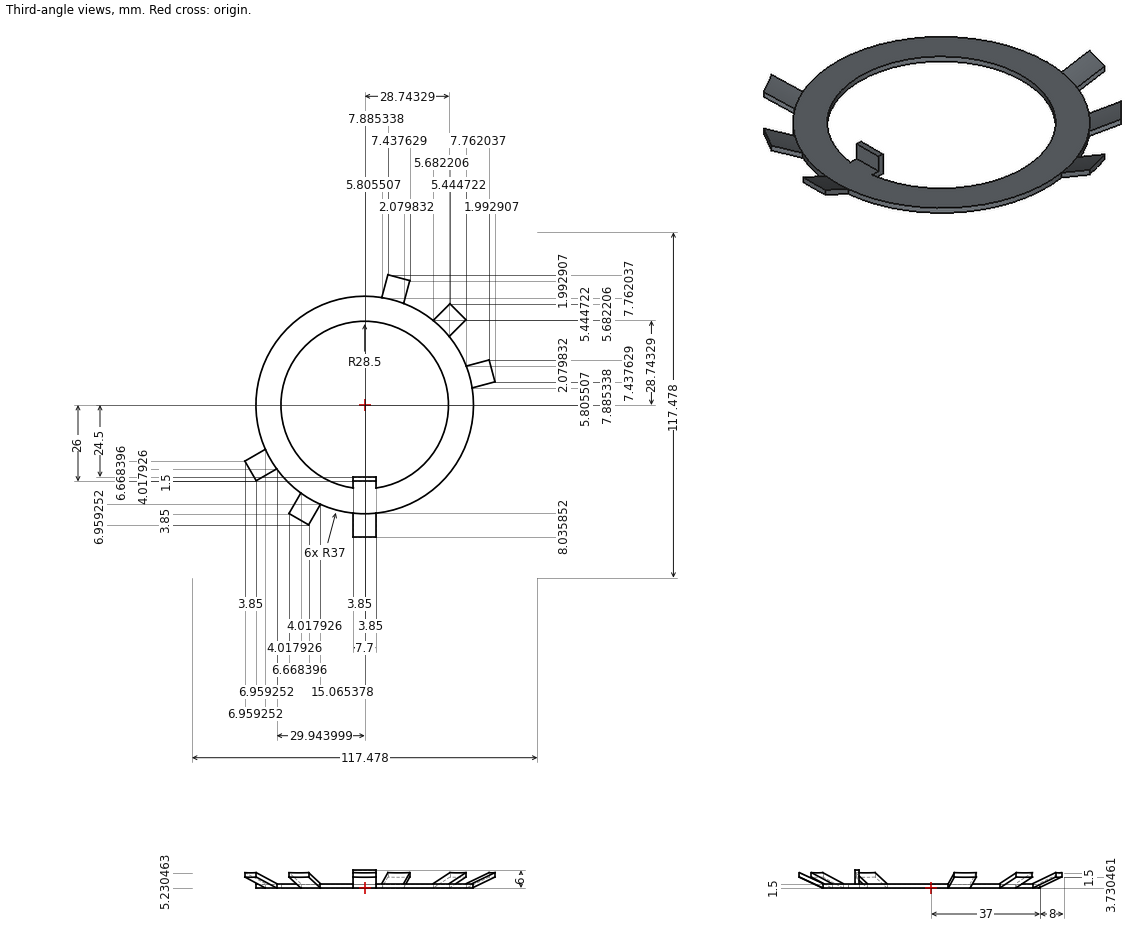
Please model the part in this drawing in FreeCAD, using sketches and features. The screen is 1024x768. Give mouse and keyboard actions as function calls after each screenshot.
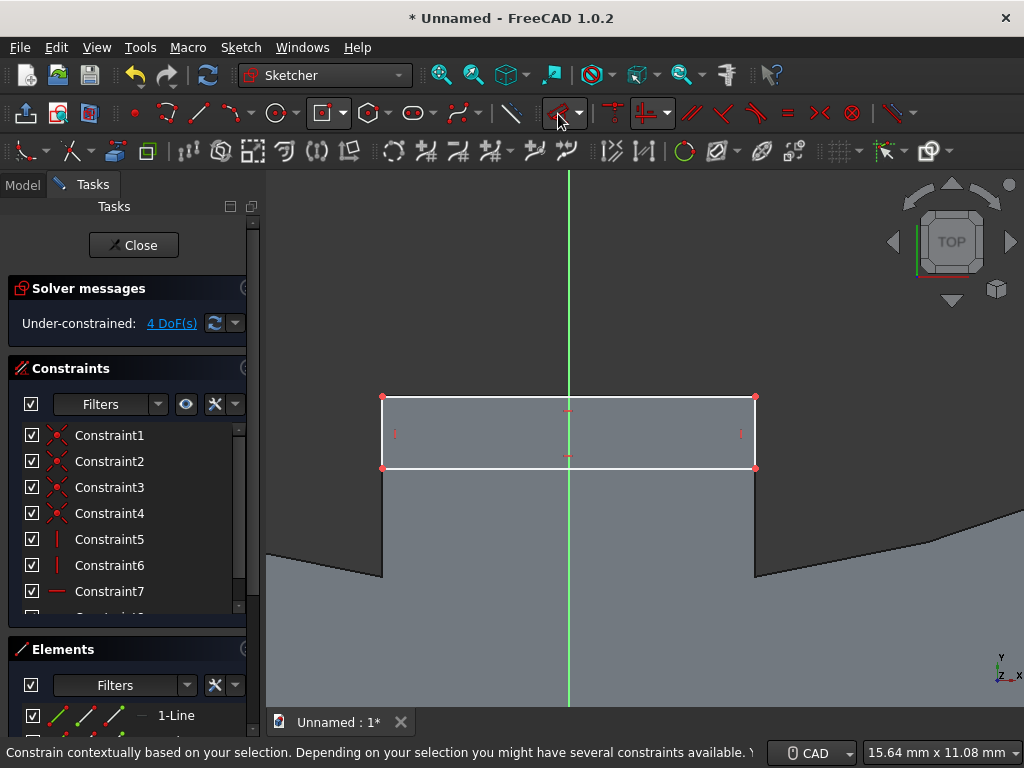
click(382, 419)
click(348, 433)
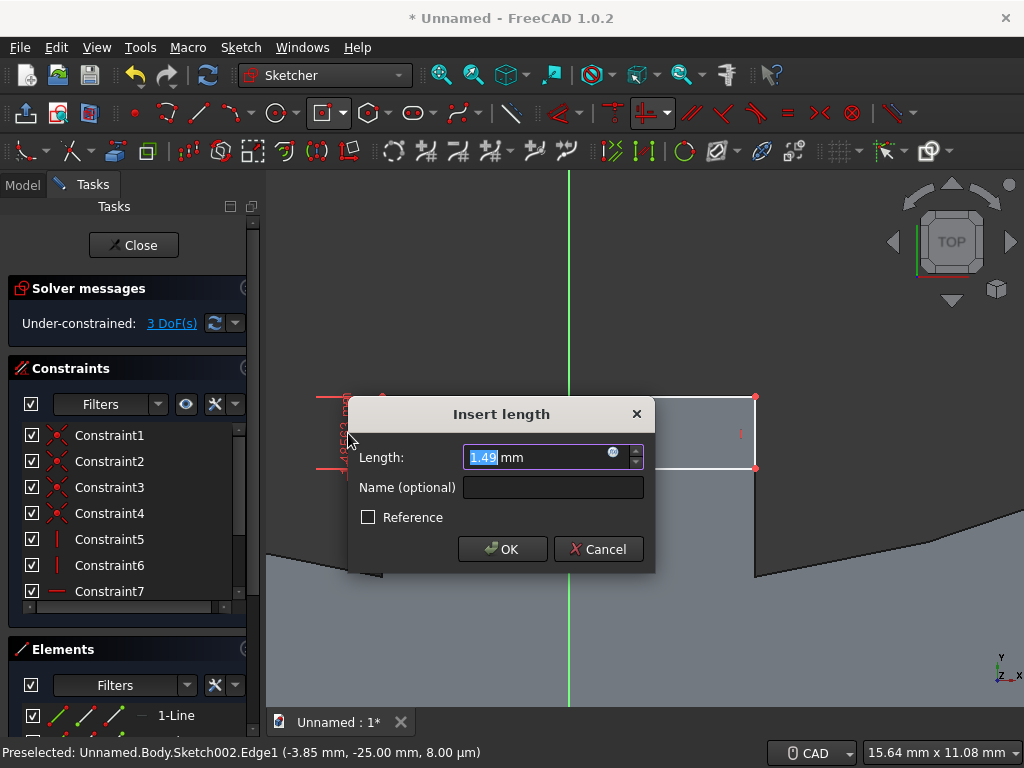
text(1.5)
key(Return)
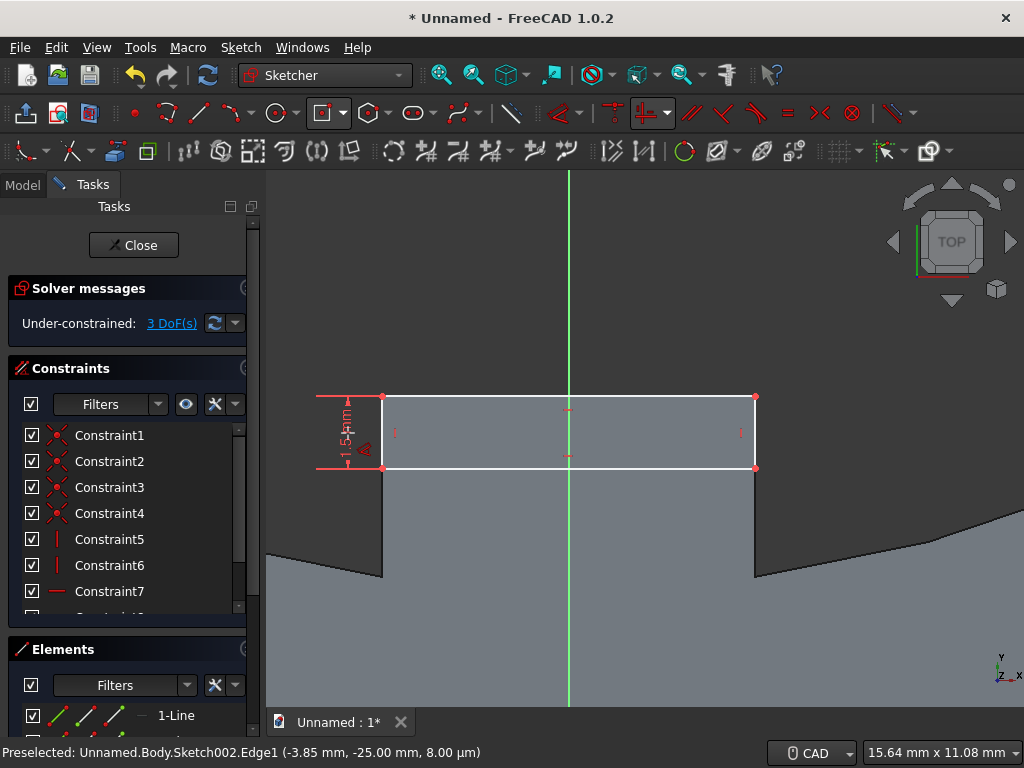
click(494, 469)
click(483, 503)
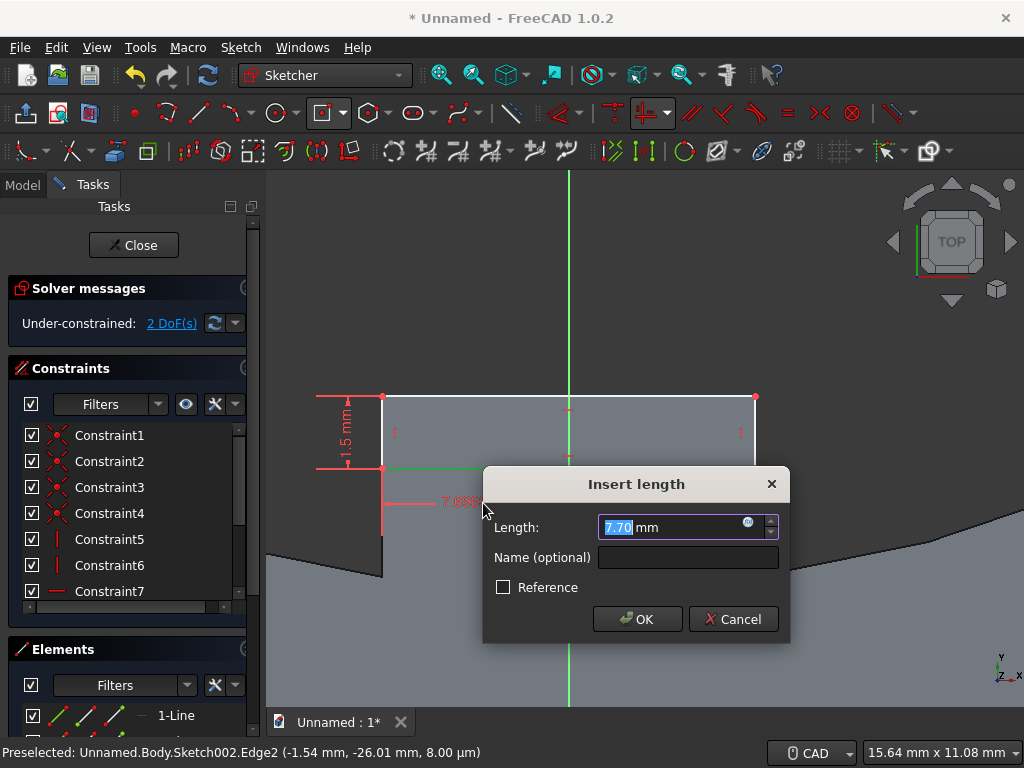
text(7.7)
key(Return)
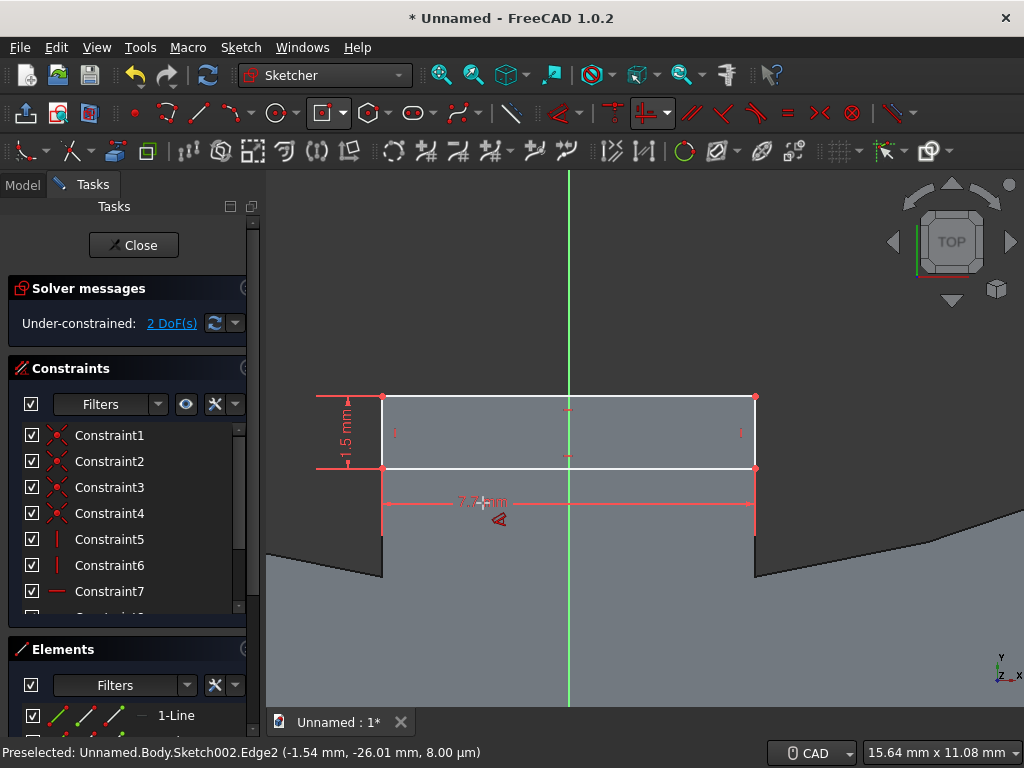
click(382, 469)
click(348, 334)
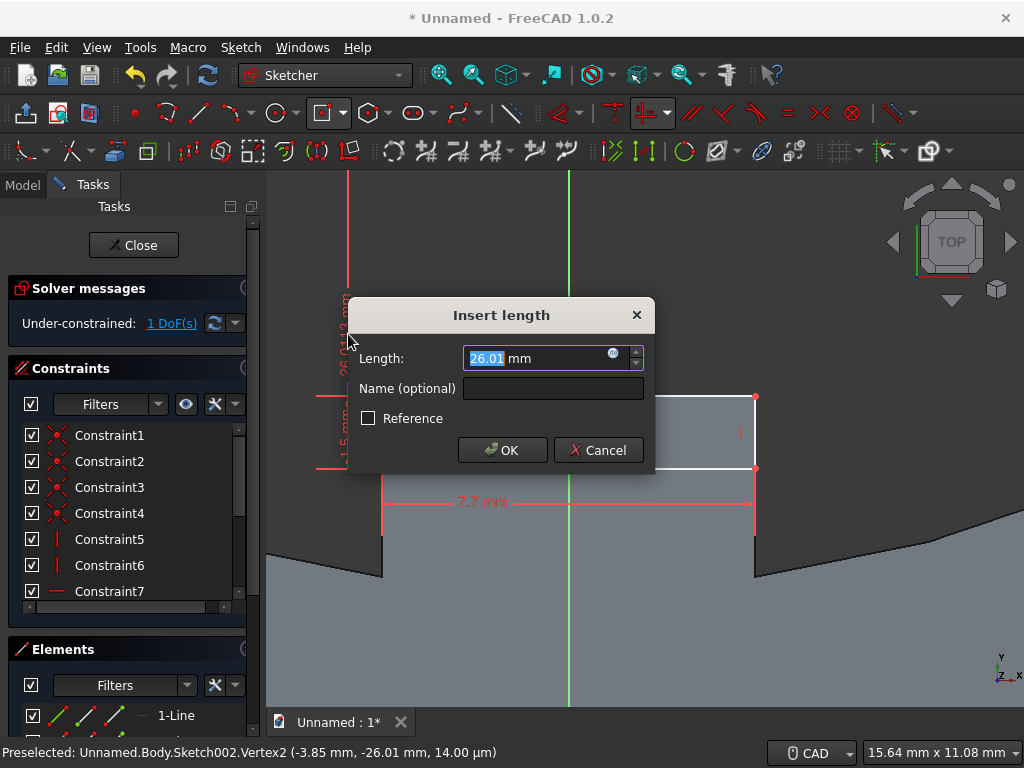
text(26)
key(Return)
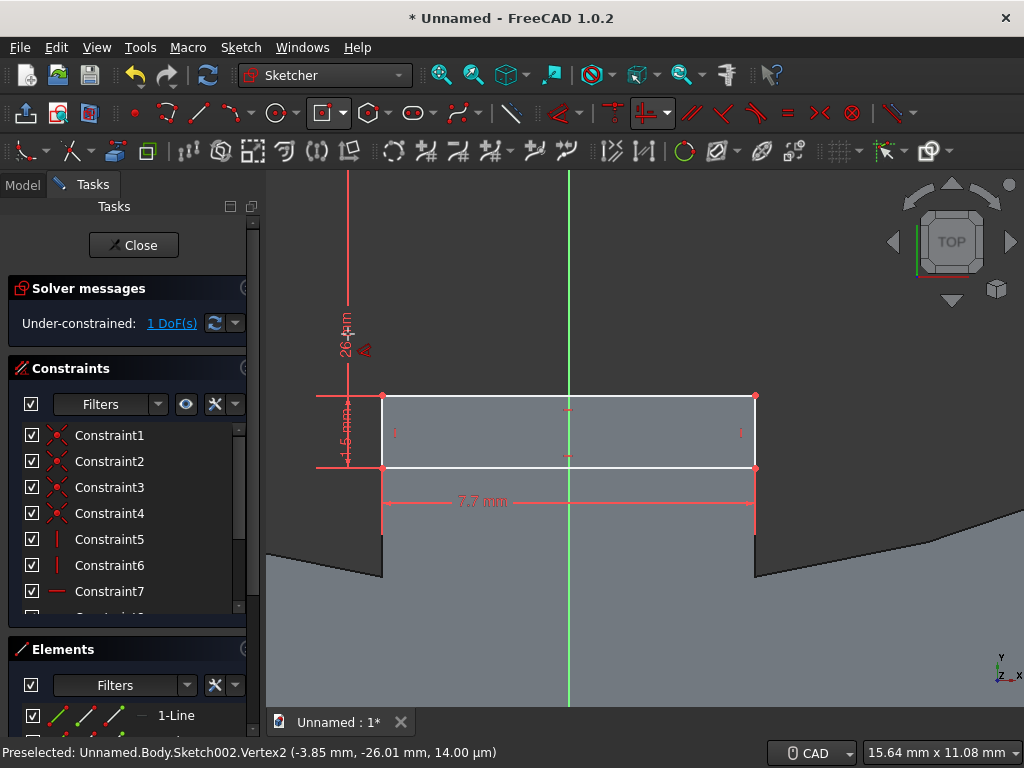
click(382, 396)
click(475, 430)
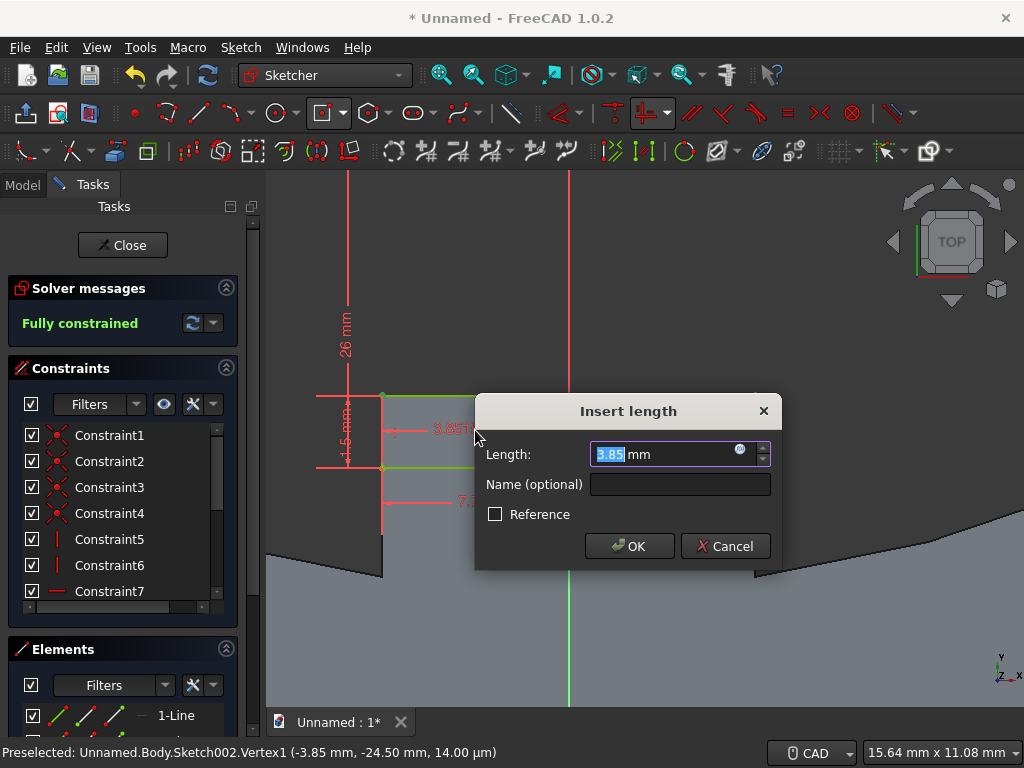
text(3.85)
key(Return)
key(Escape)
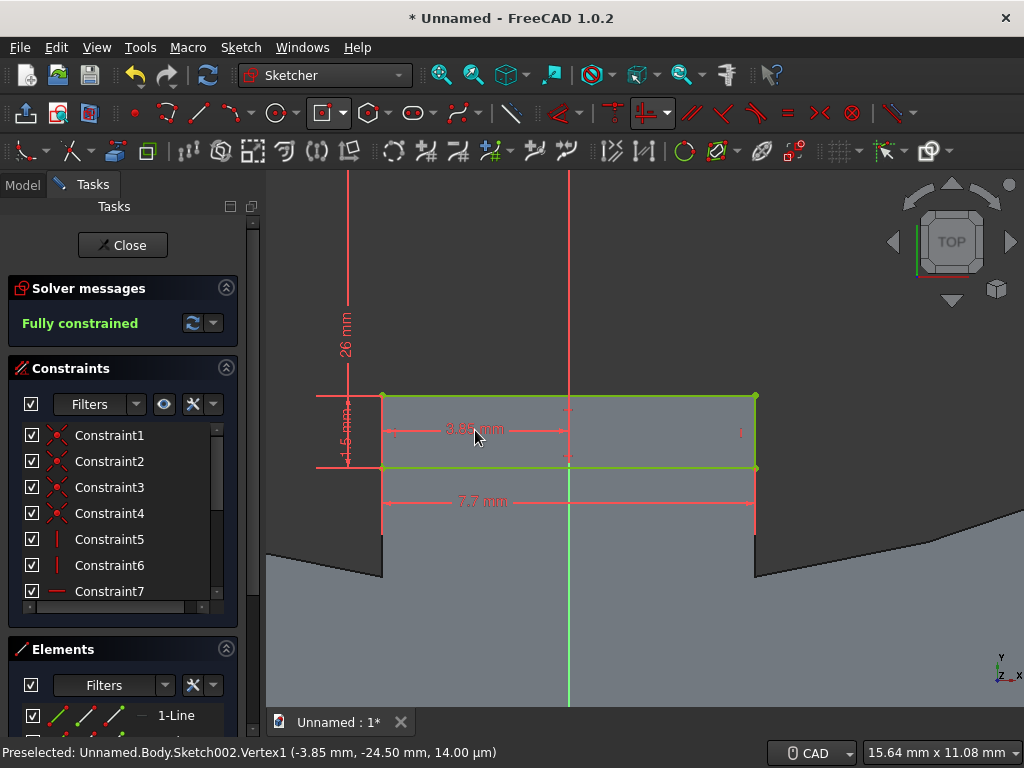
click(123, 245)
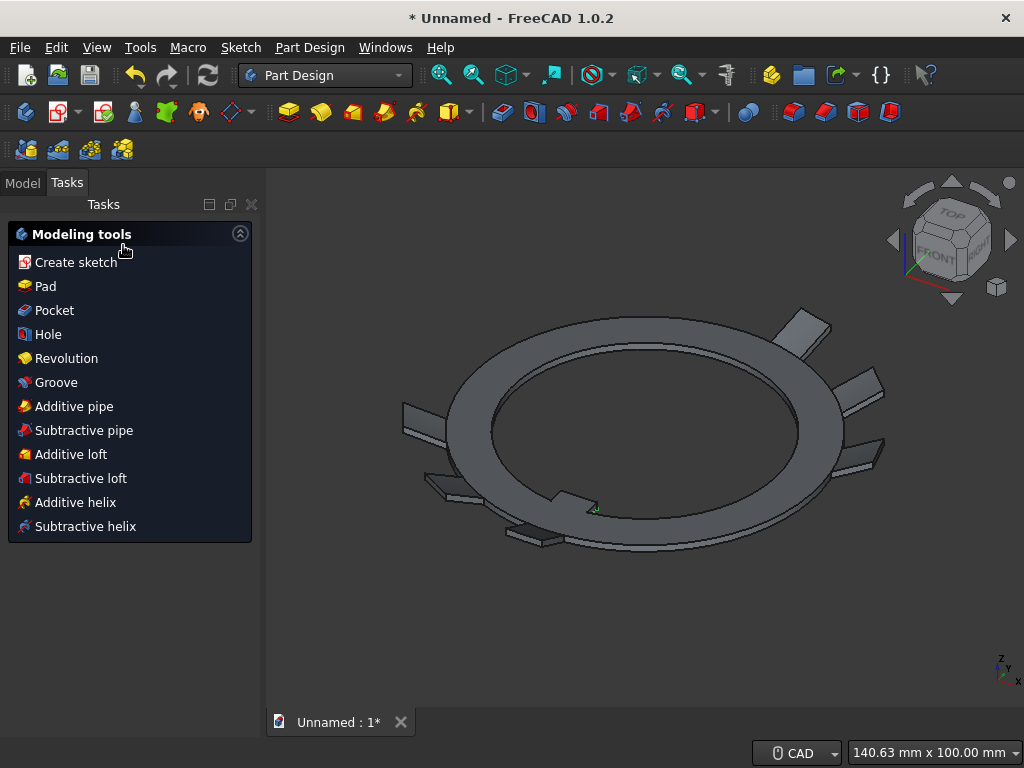
click(290, 112)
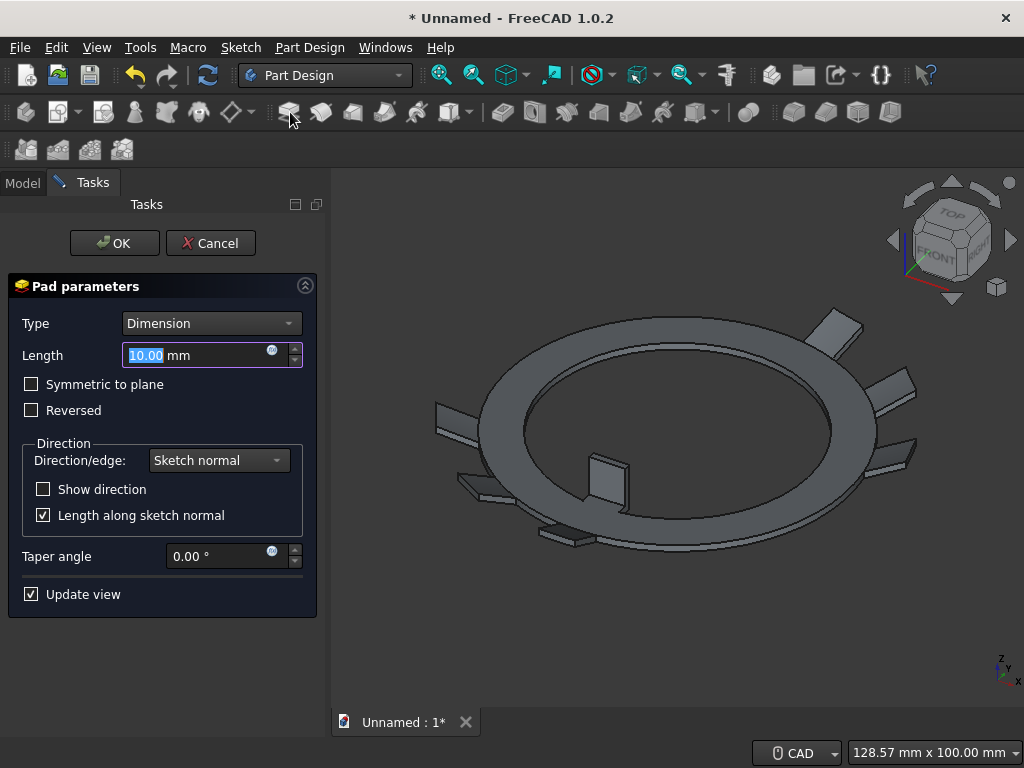
text(6)
key(Tab)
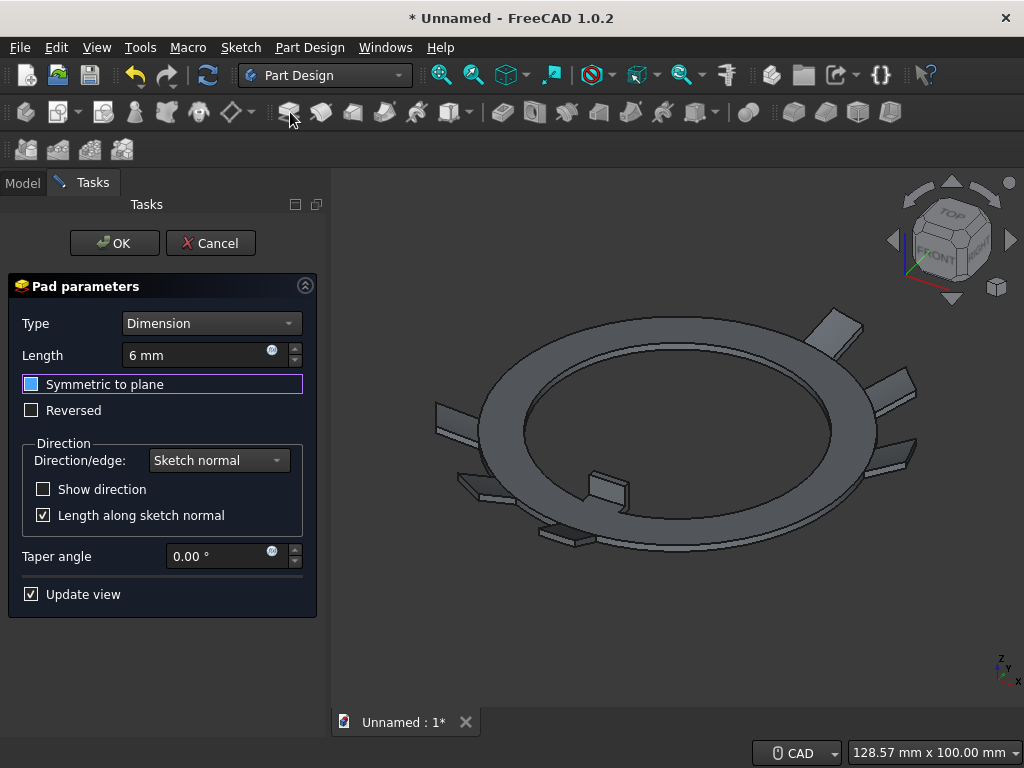
click(115, 243)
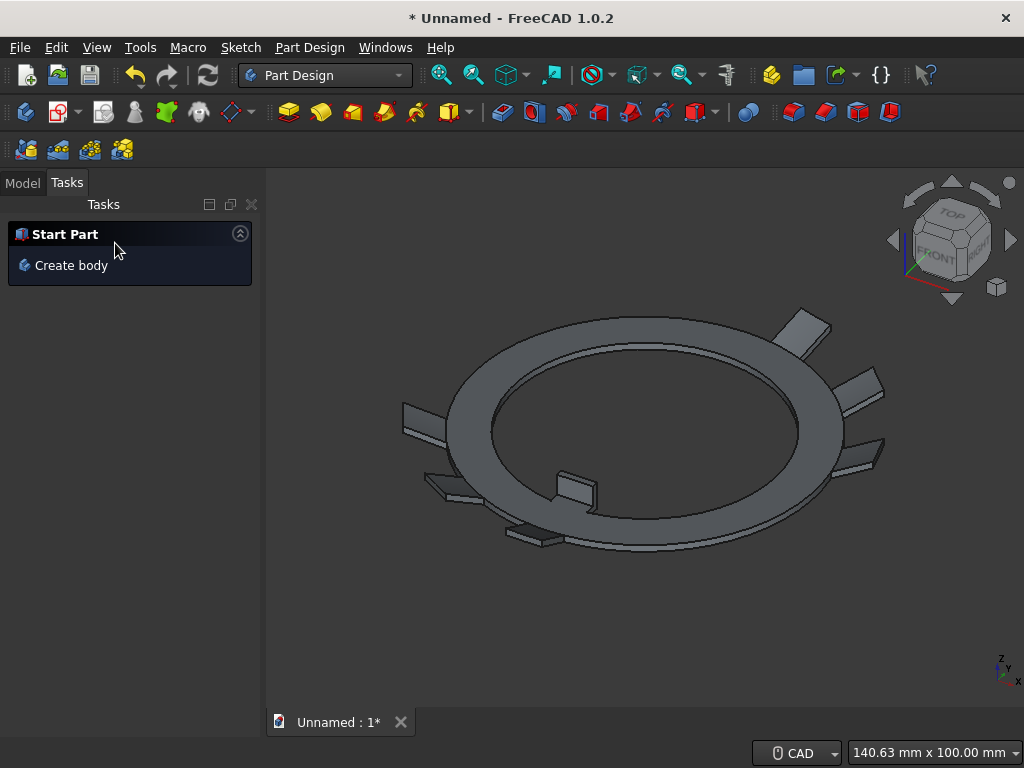
key(0)